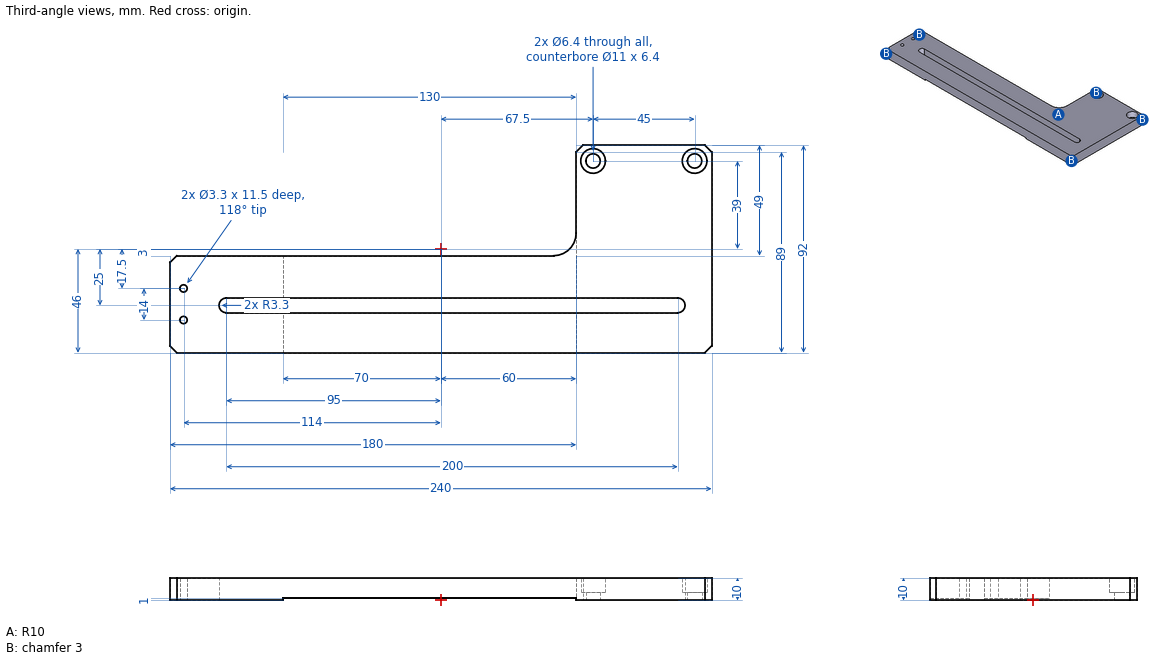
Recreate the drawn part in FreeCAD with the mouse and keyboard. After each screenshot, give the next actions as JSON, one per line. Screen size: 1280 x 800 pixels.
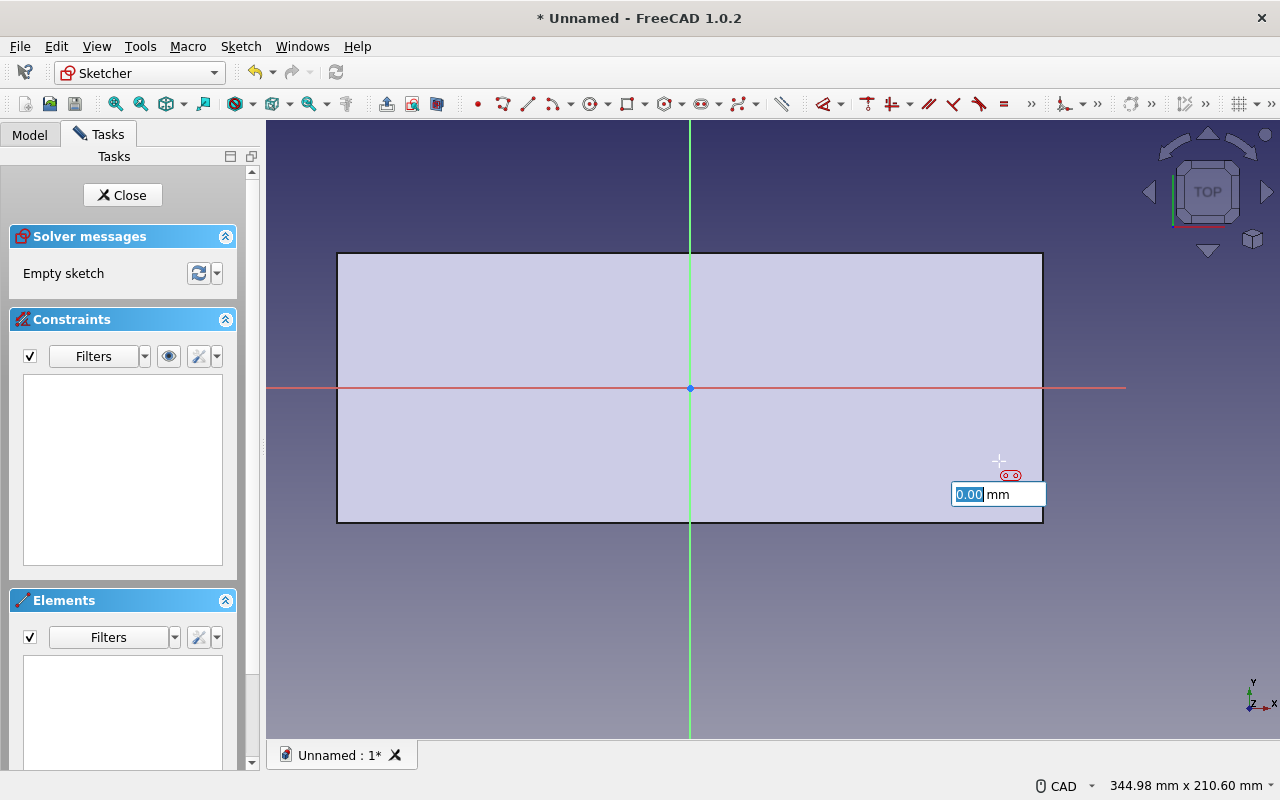
{"action": "scroll", "coordinate": [705, 452], "scroll_direction": "up", "scroll_amount": 3}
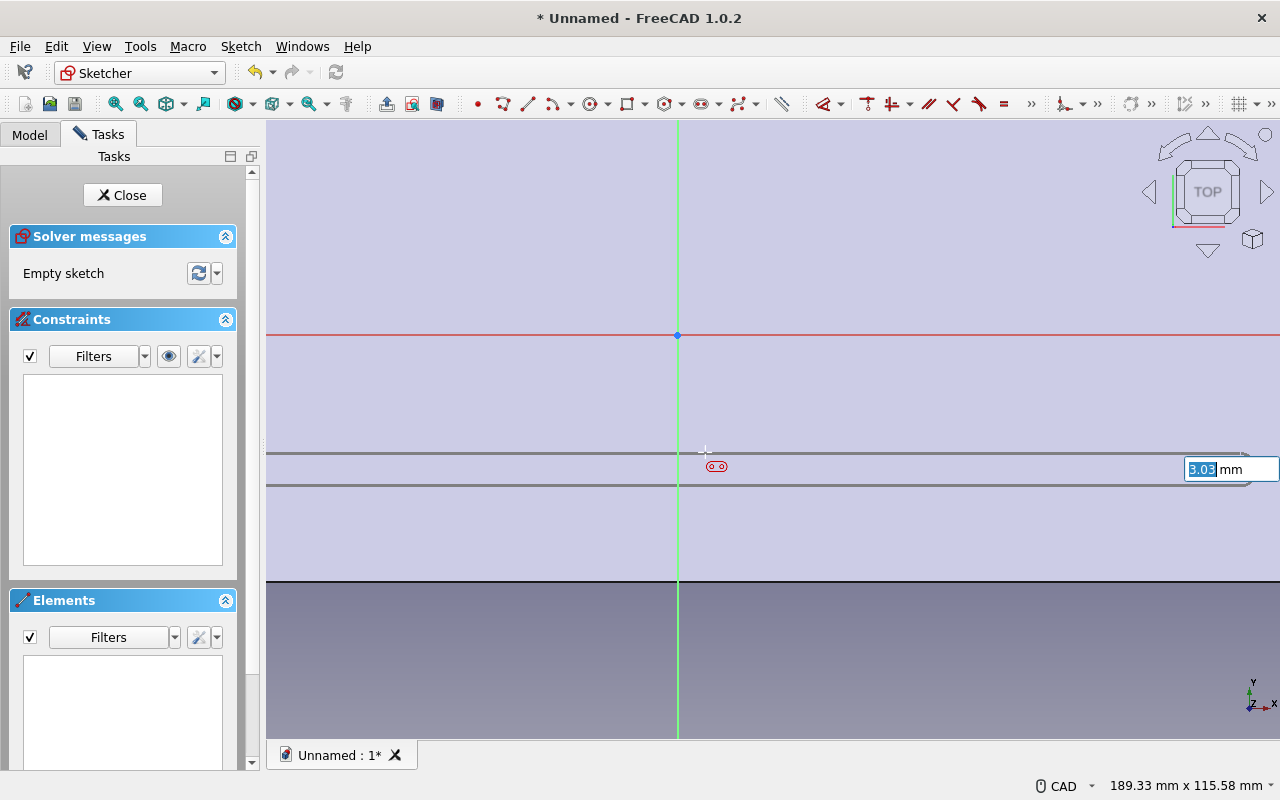
{"action": "left_click", "coordinate": [704, 451]}
{"action": "key", "text": "Escape"}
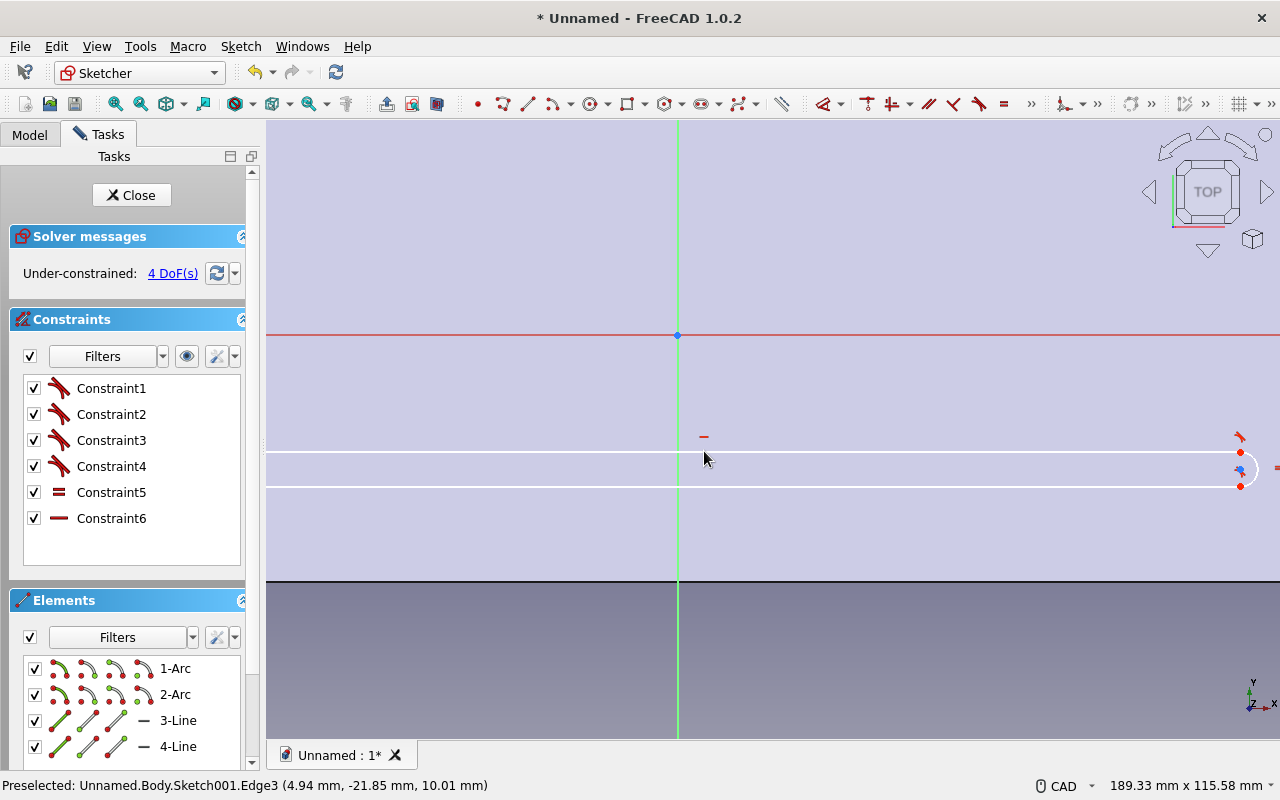
{"action": "scroll", "coordinate": [705, 452], "scroll_direction": "down", "scroll_amount": 3}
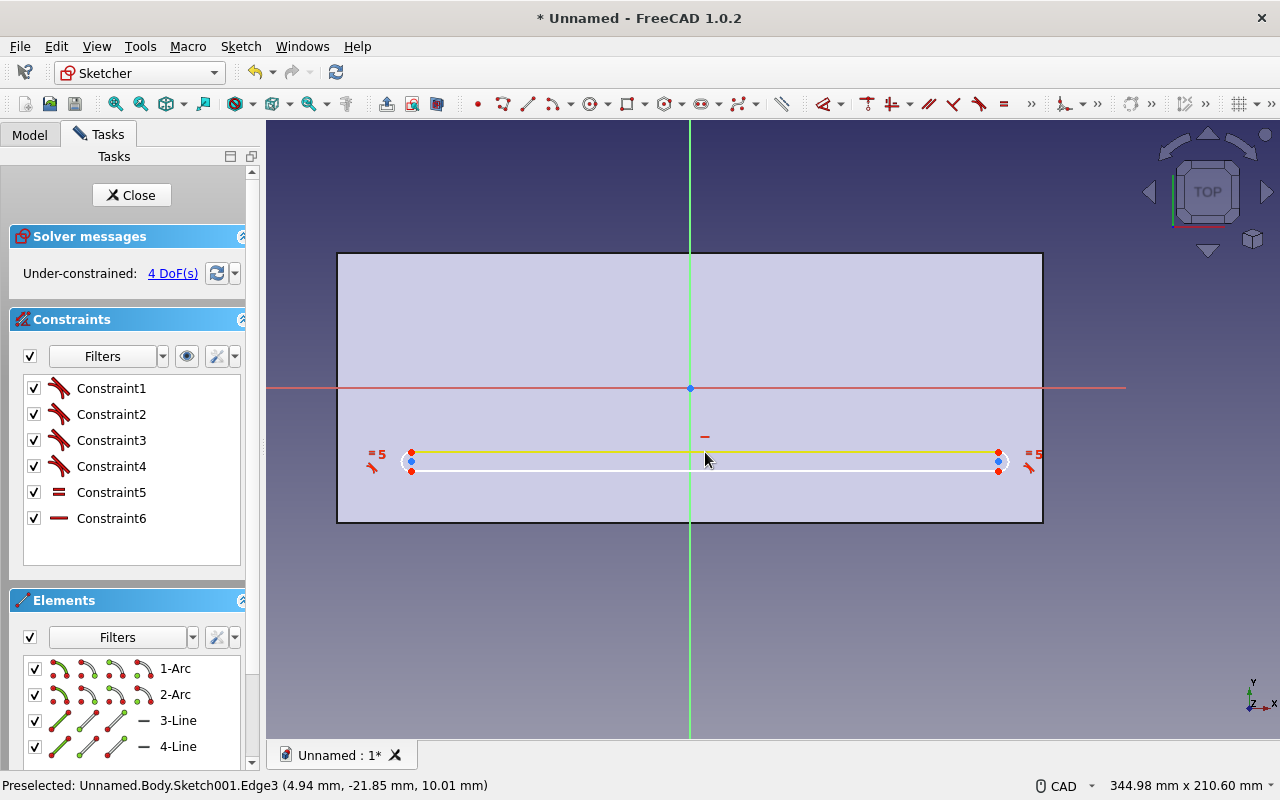
{"action": "scroll", "coordinate": [403, 456], "scroll_direction": "up", "scroll_amount": 8}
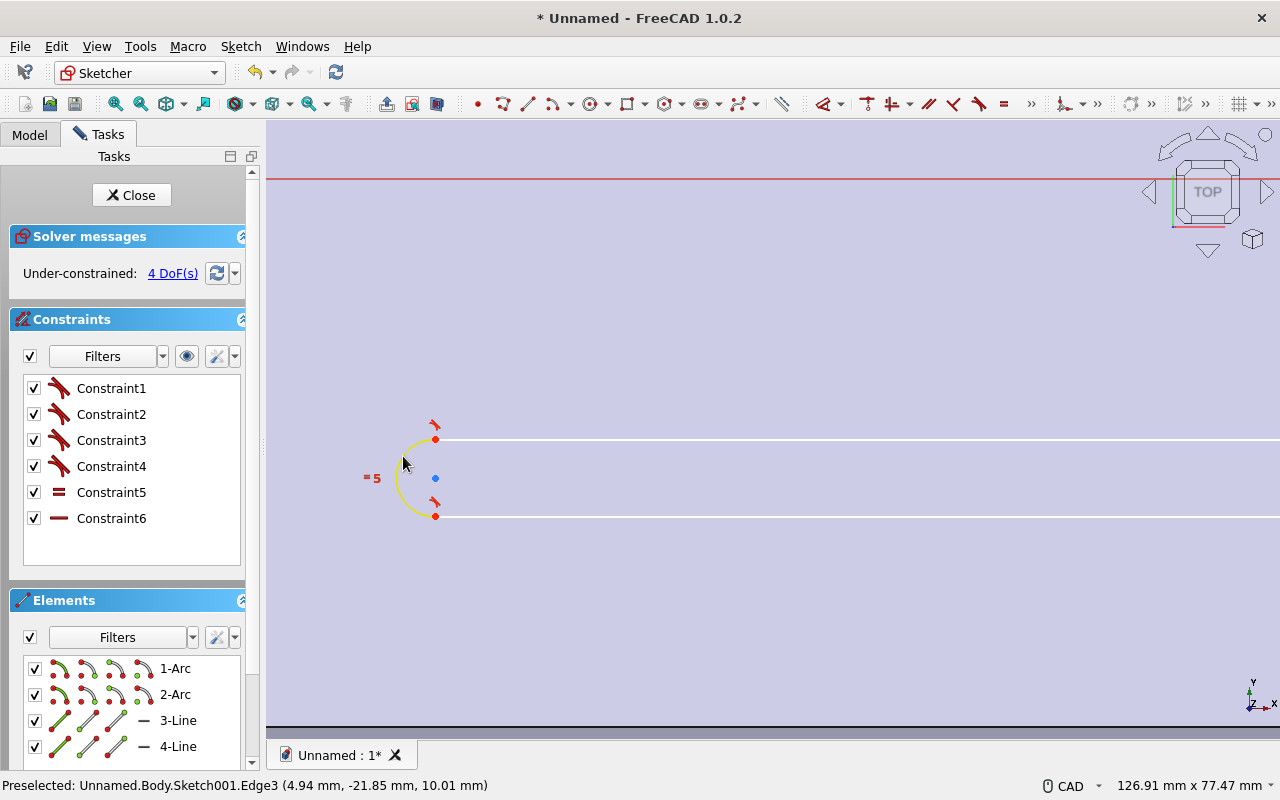
{"action": "left_click", "coordinate": [404, 455]}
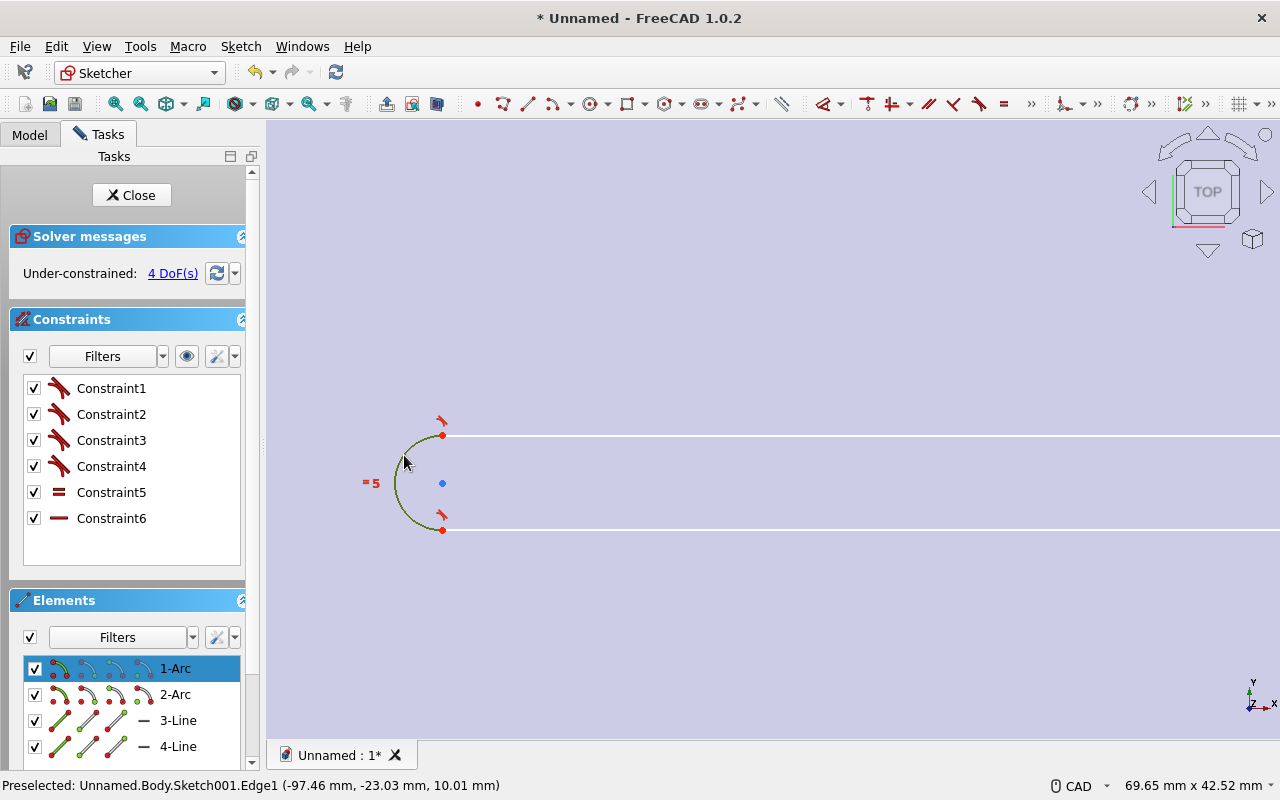
{"action": "key", "text": "k r"}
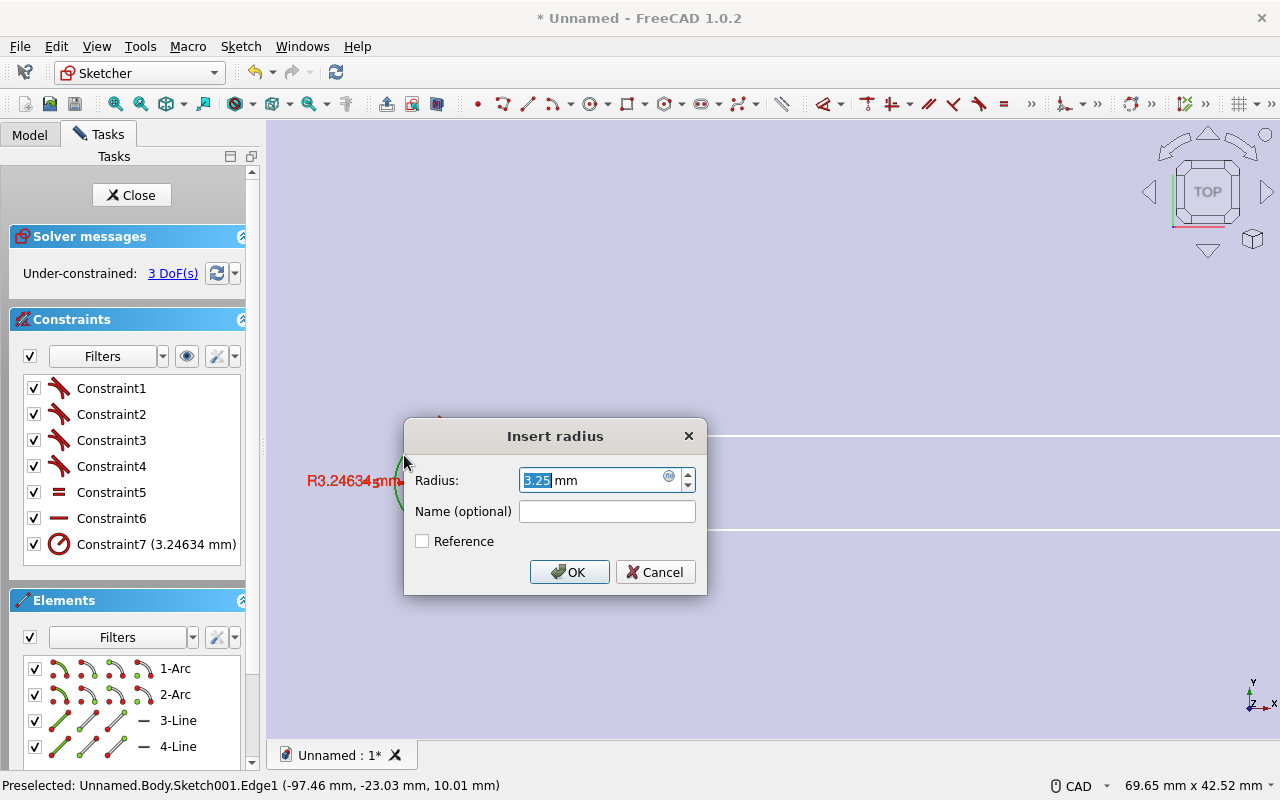
{"action": "type", "text": "3.3"}
{"action": "key", "text": "Return"}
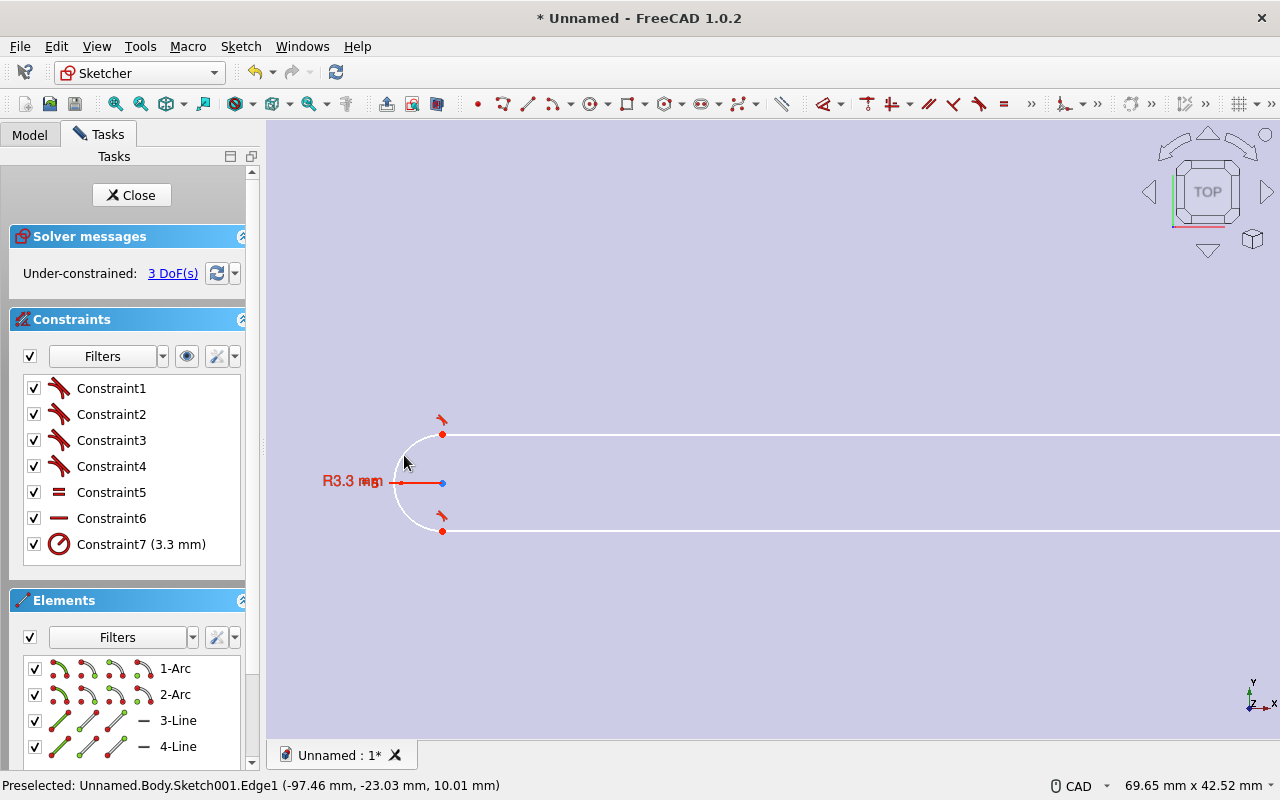
{"action": "scroll", "coordinate": [403, 456], "scroll_direction": "down", "scroll_amount": 8}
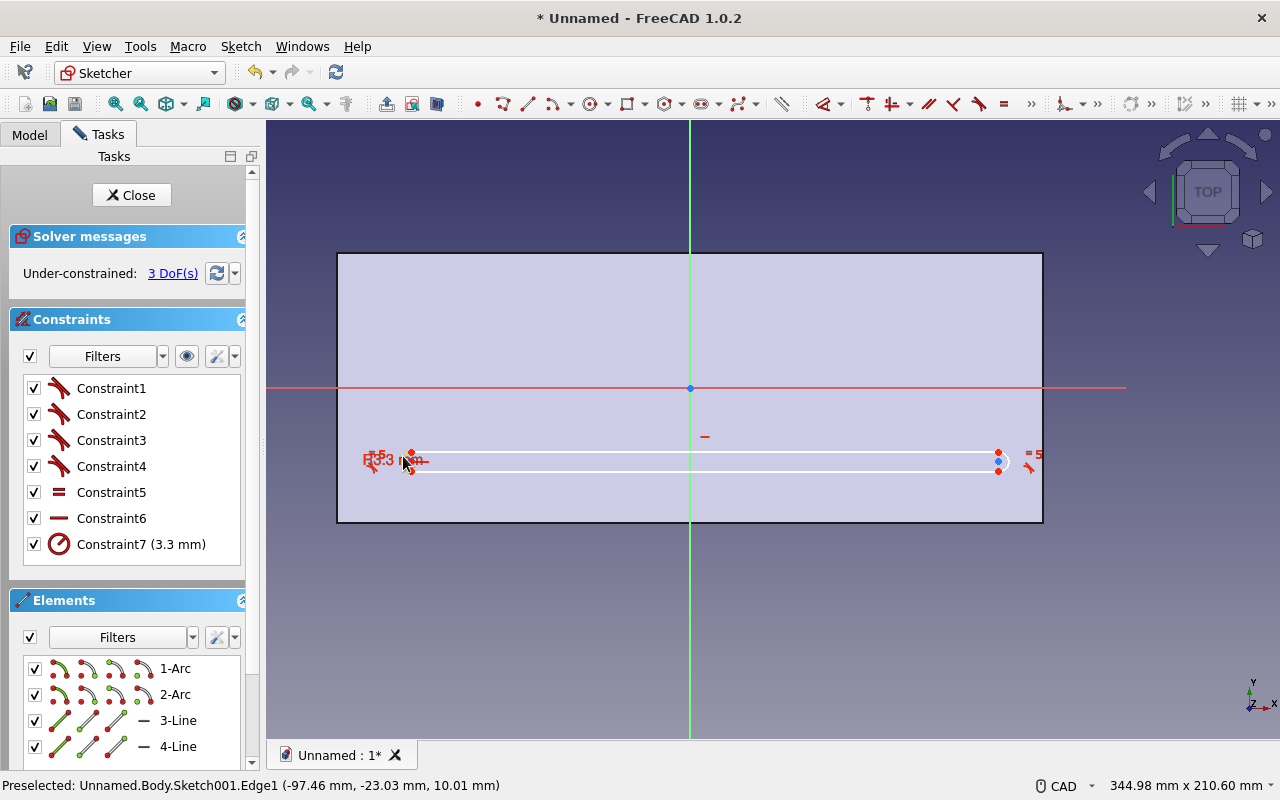
{"action": "left_click", "coordinate": [529, 452]}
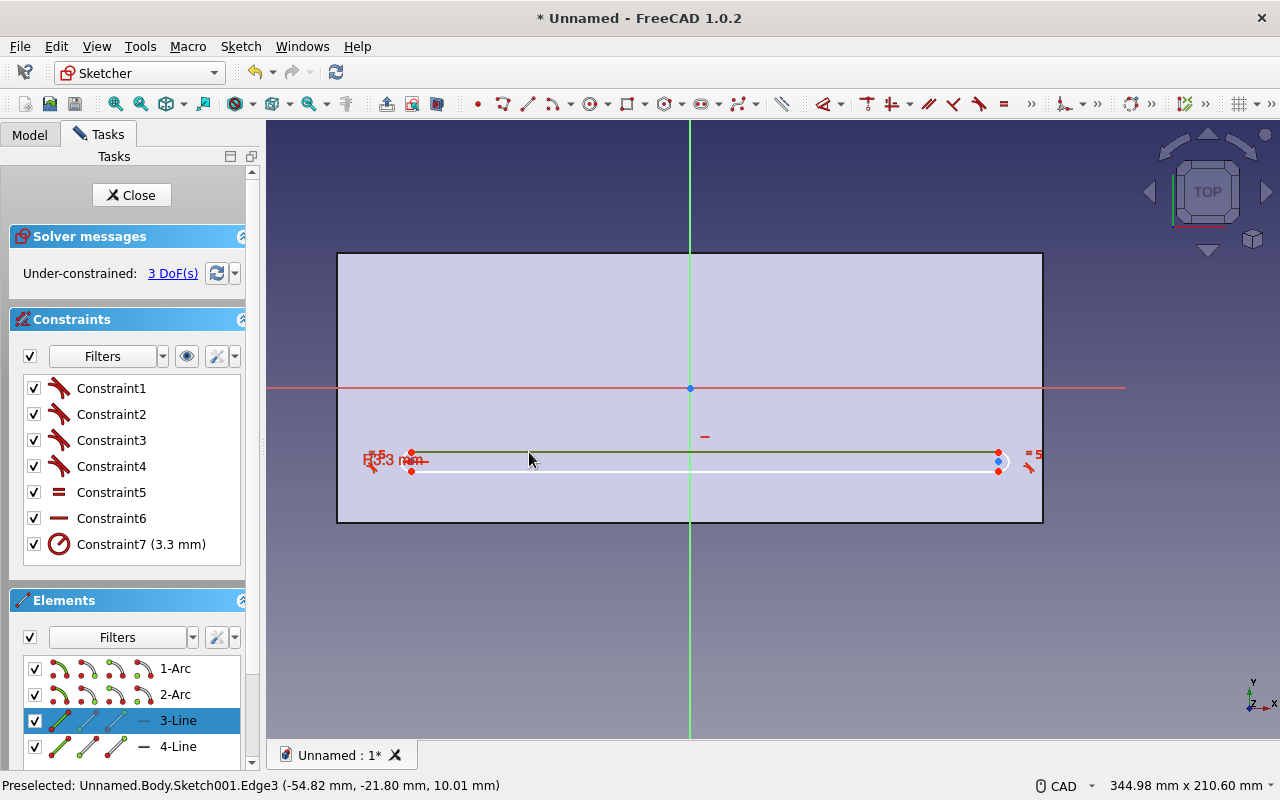
{"action": "key", "text": "l"}